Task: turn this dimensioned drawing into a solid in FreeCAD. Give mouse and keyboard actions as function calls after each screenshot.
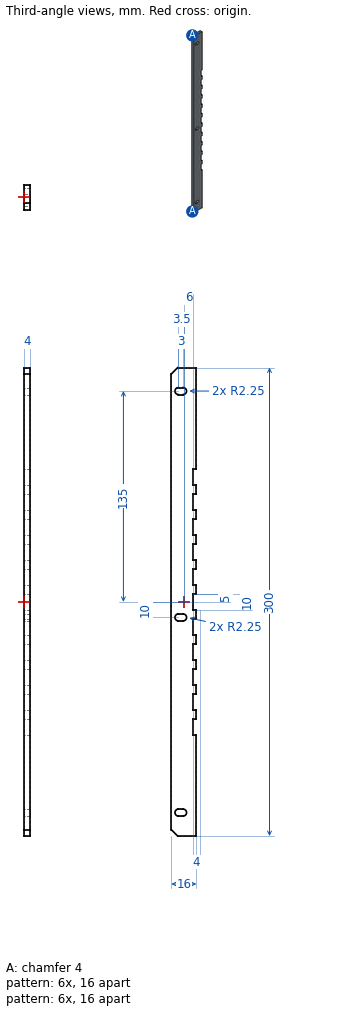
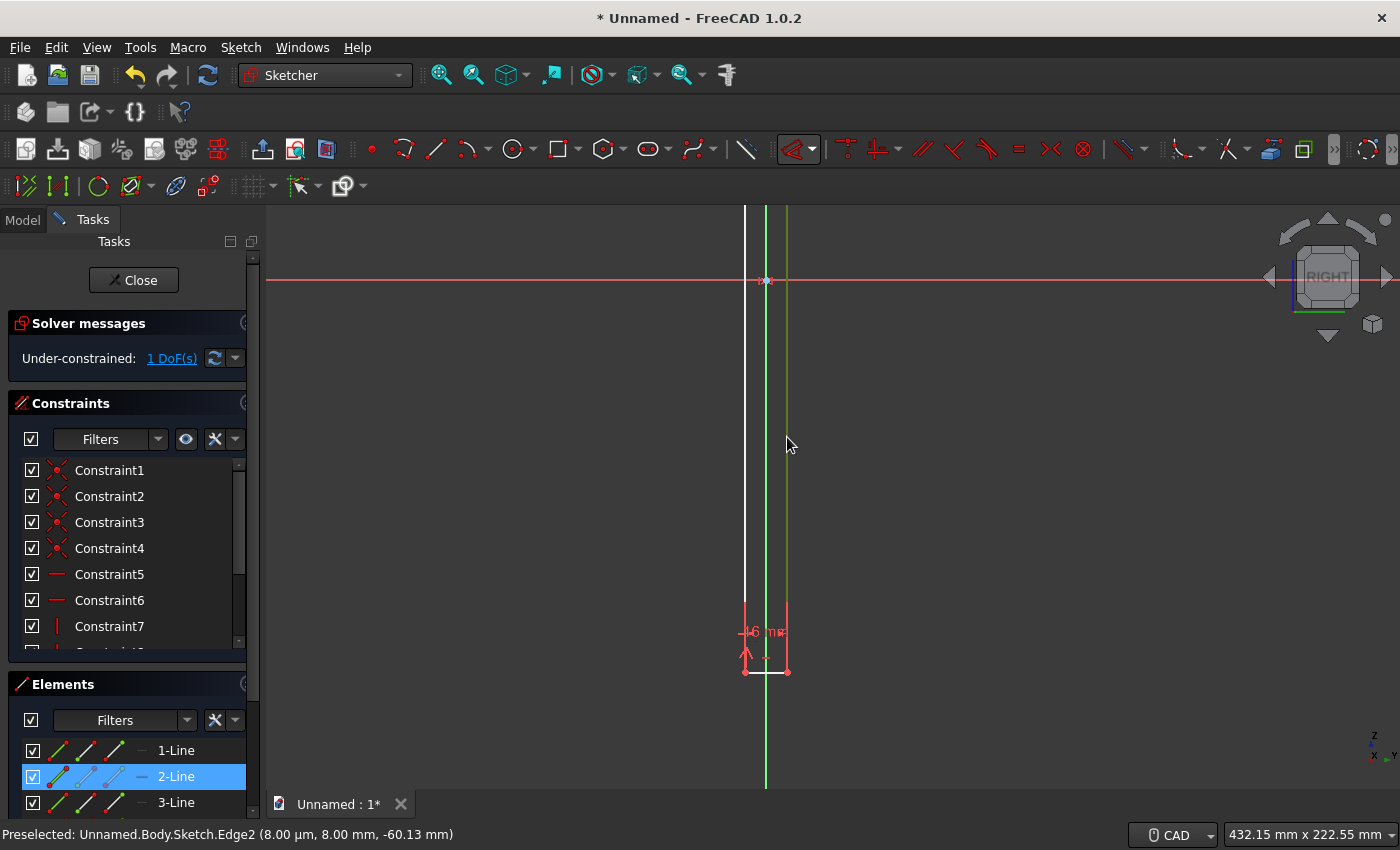
key(i)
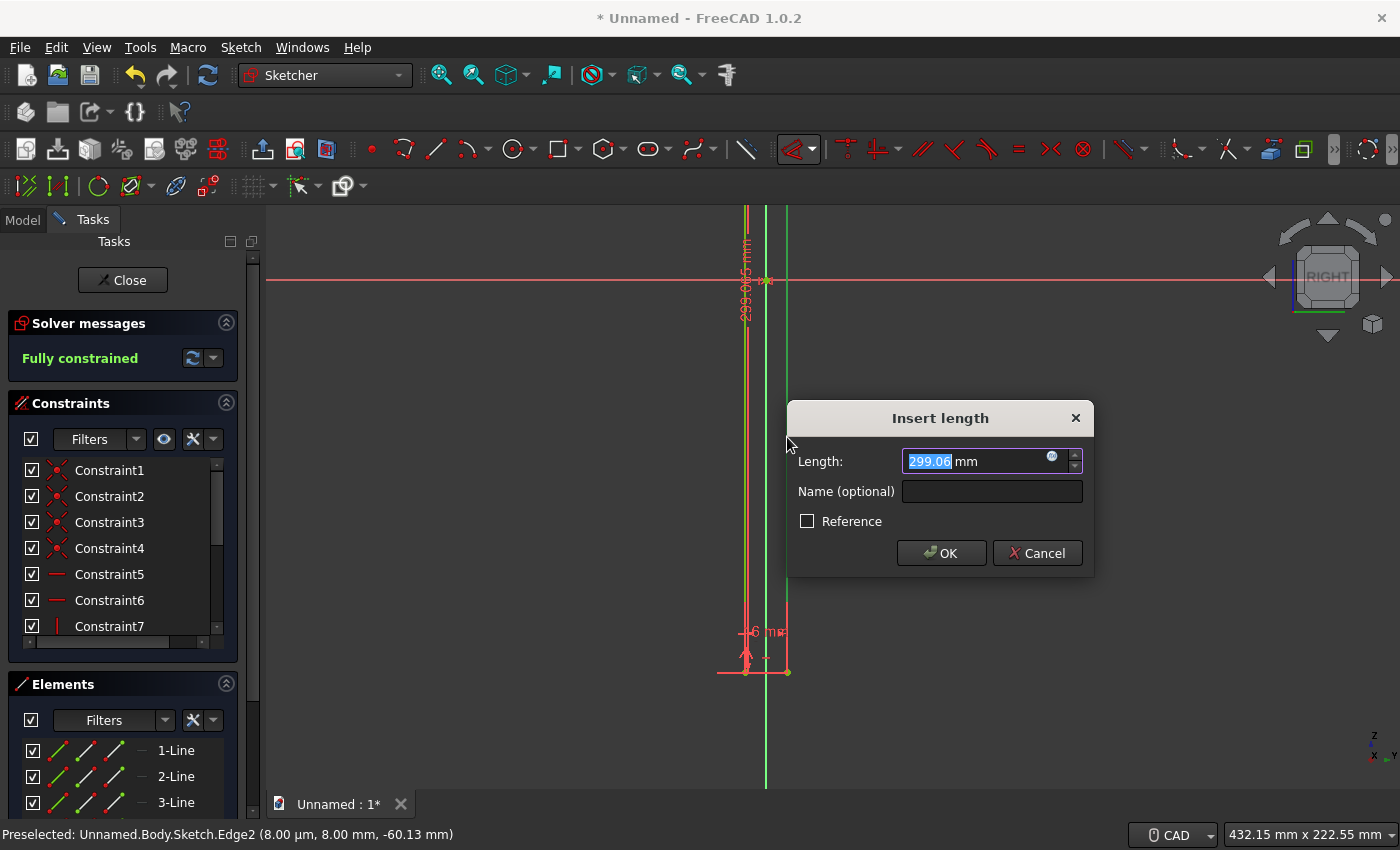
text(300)
key(Return)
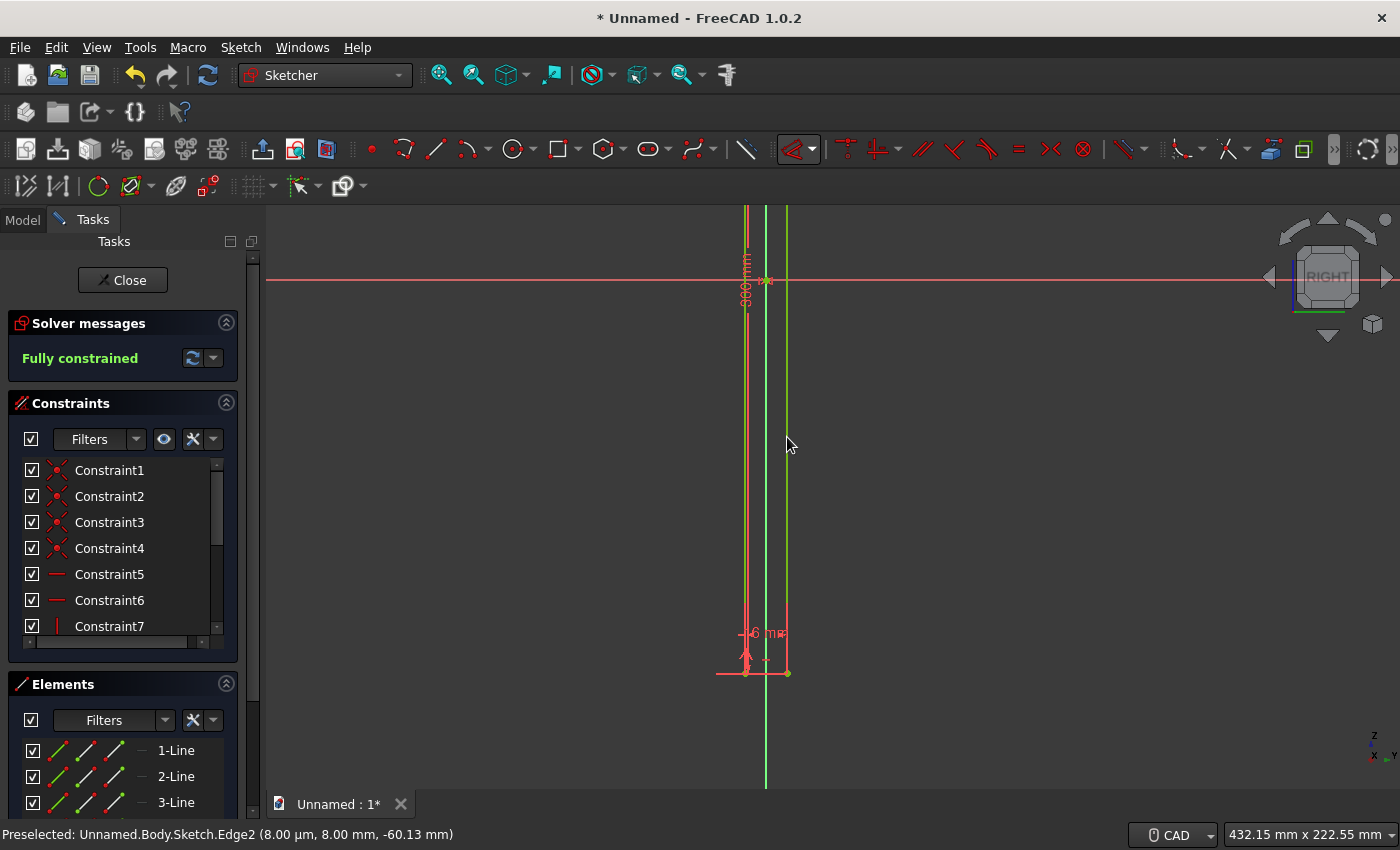
click(123, 280)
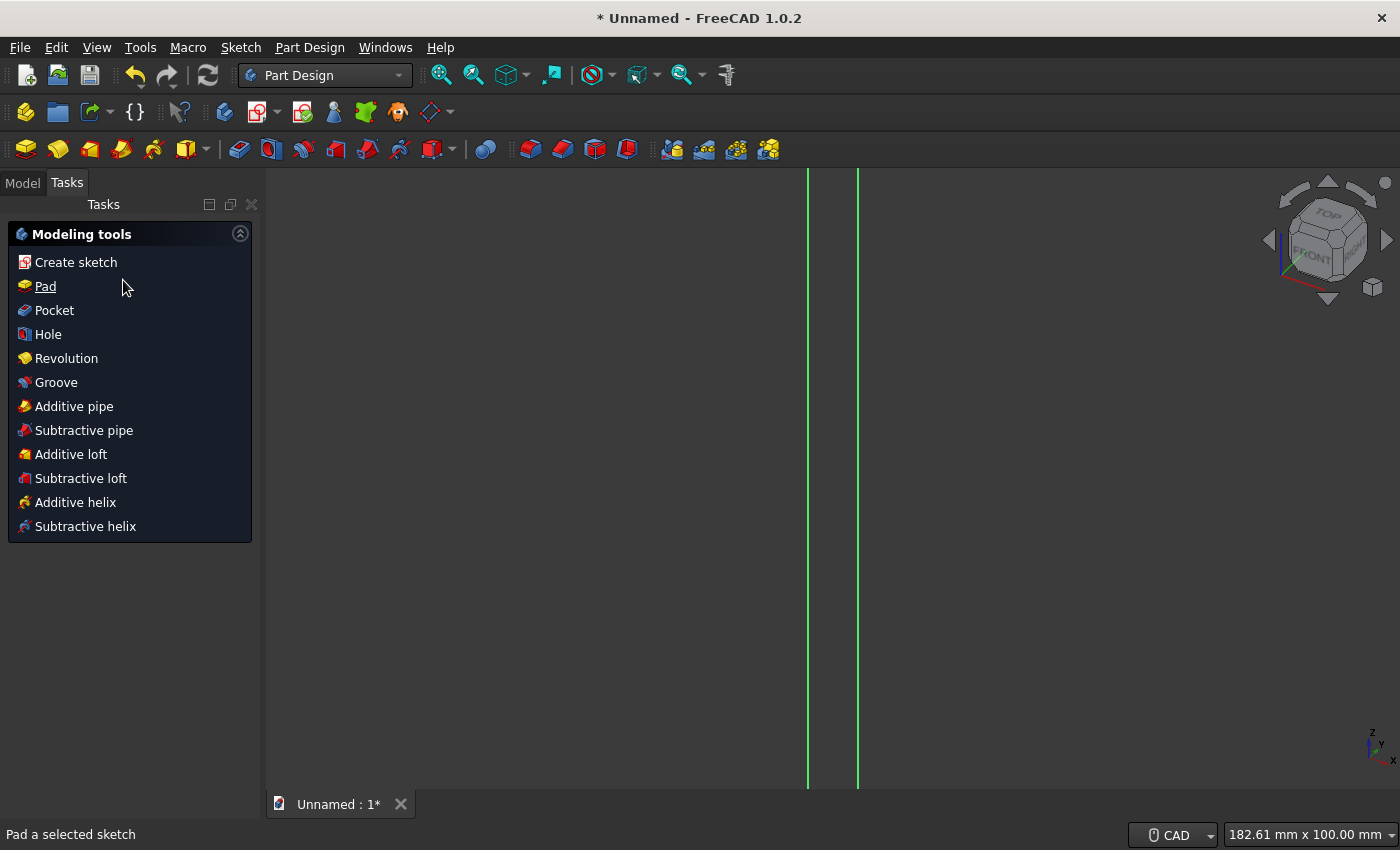
click(26, 150)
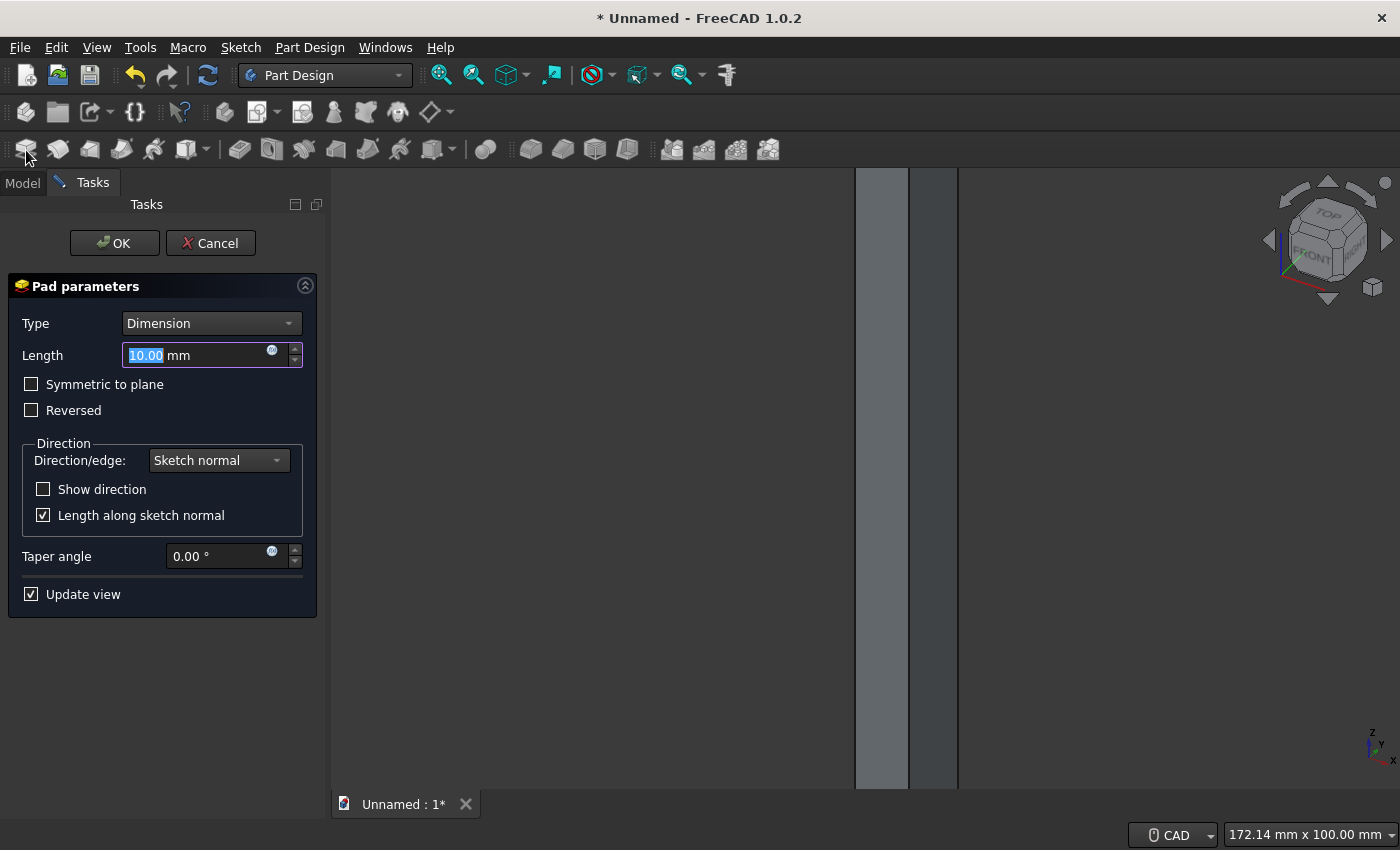
text(4)
key(Tab)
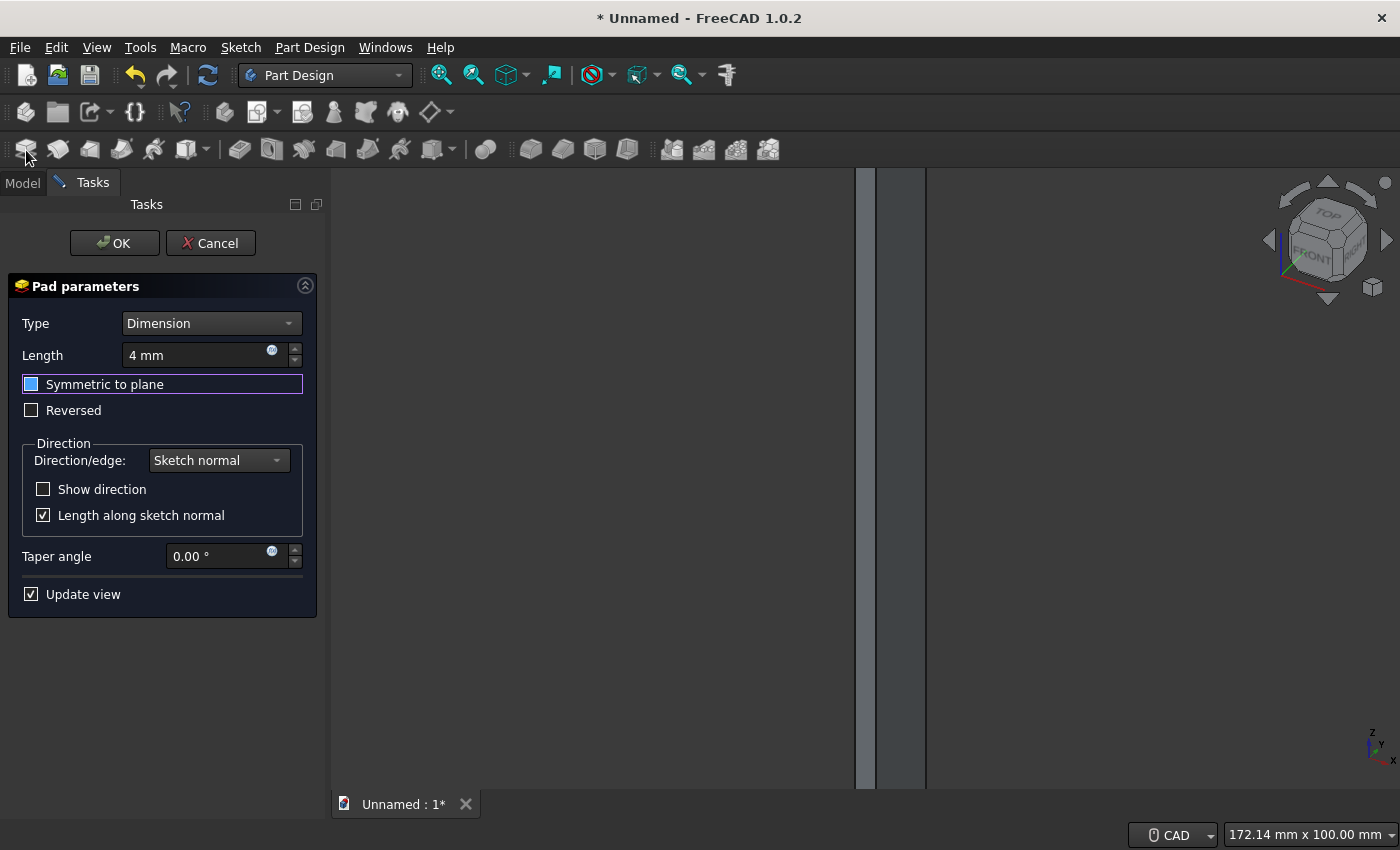
click(115, 243)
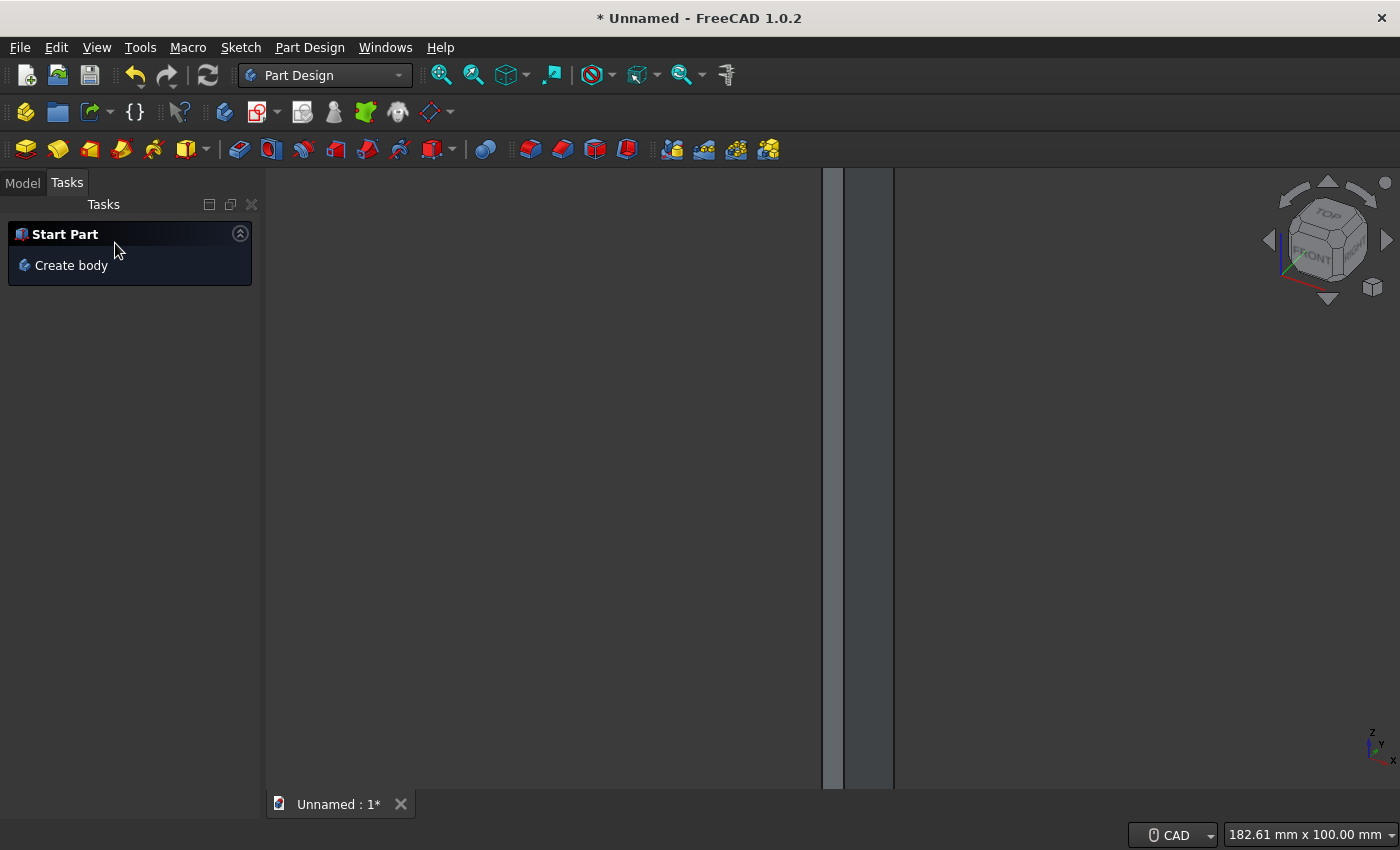
click(442, 76)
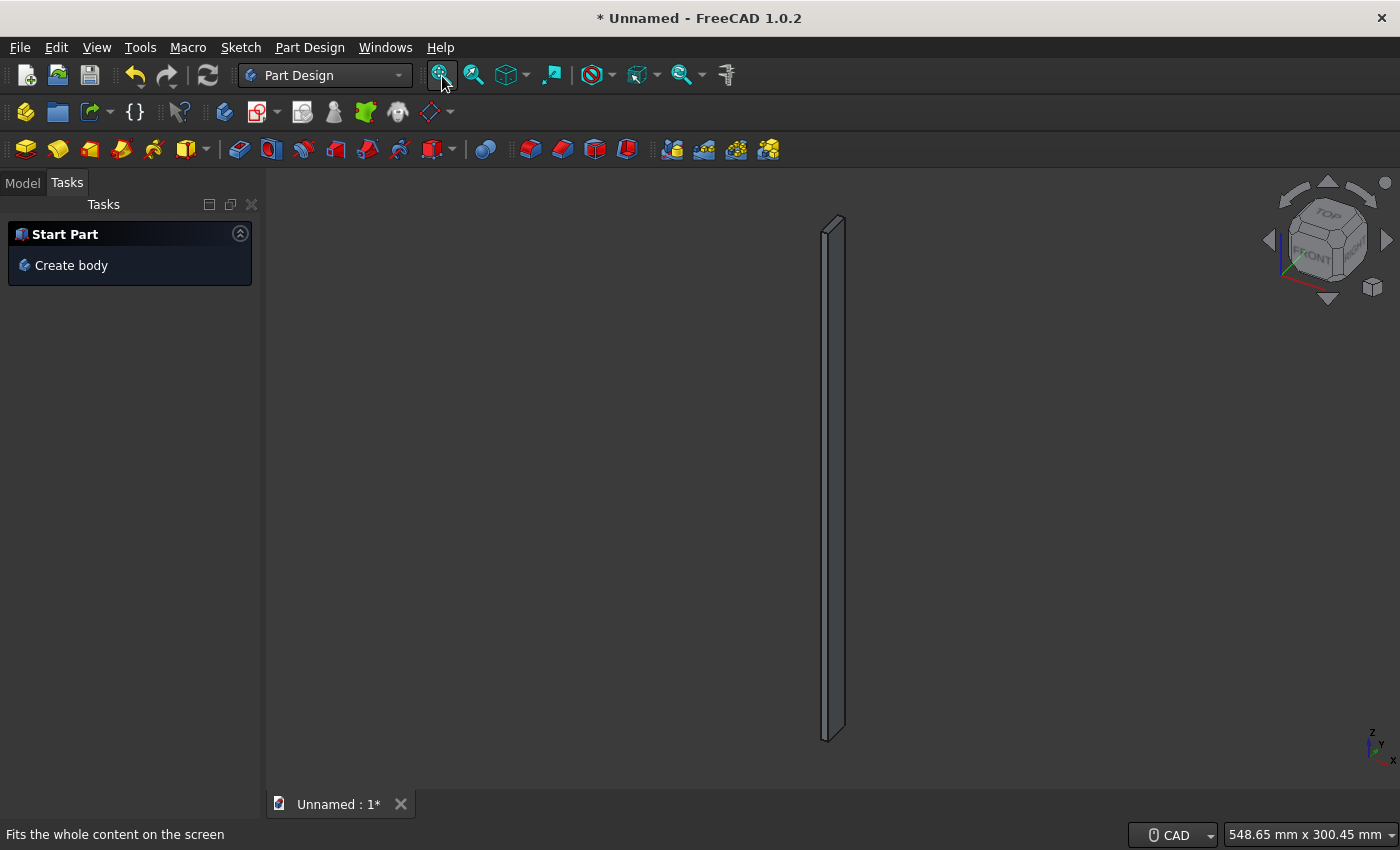
scroll(825, 740, up, 8)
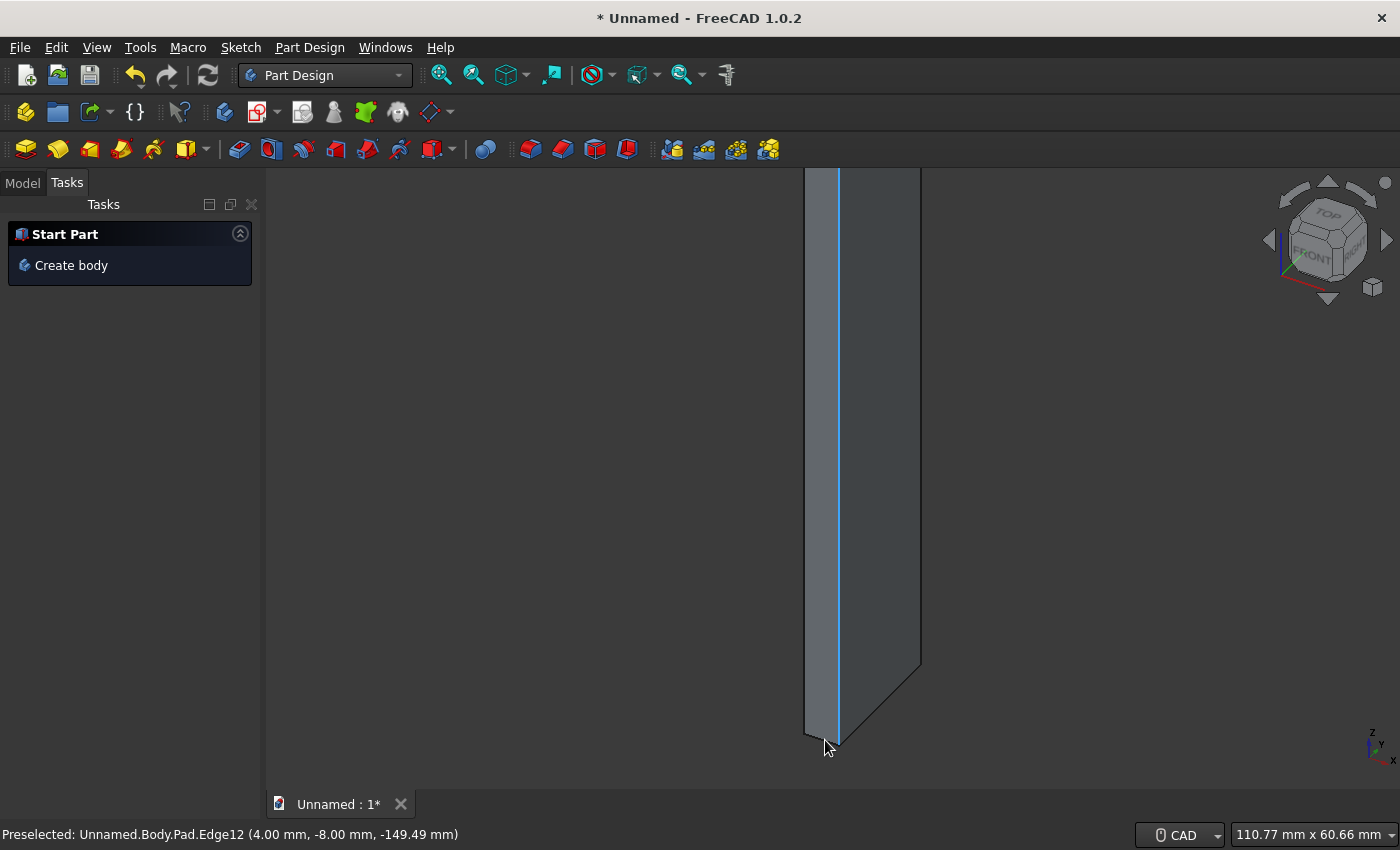
click(442, 76)